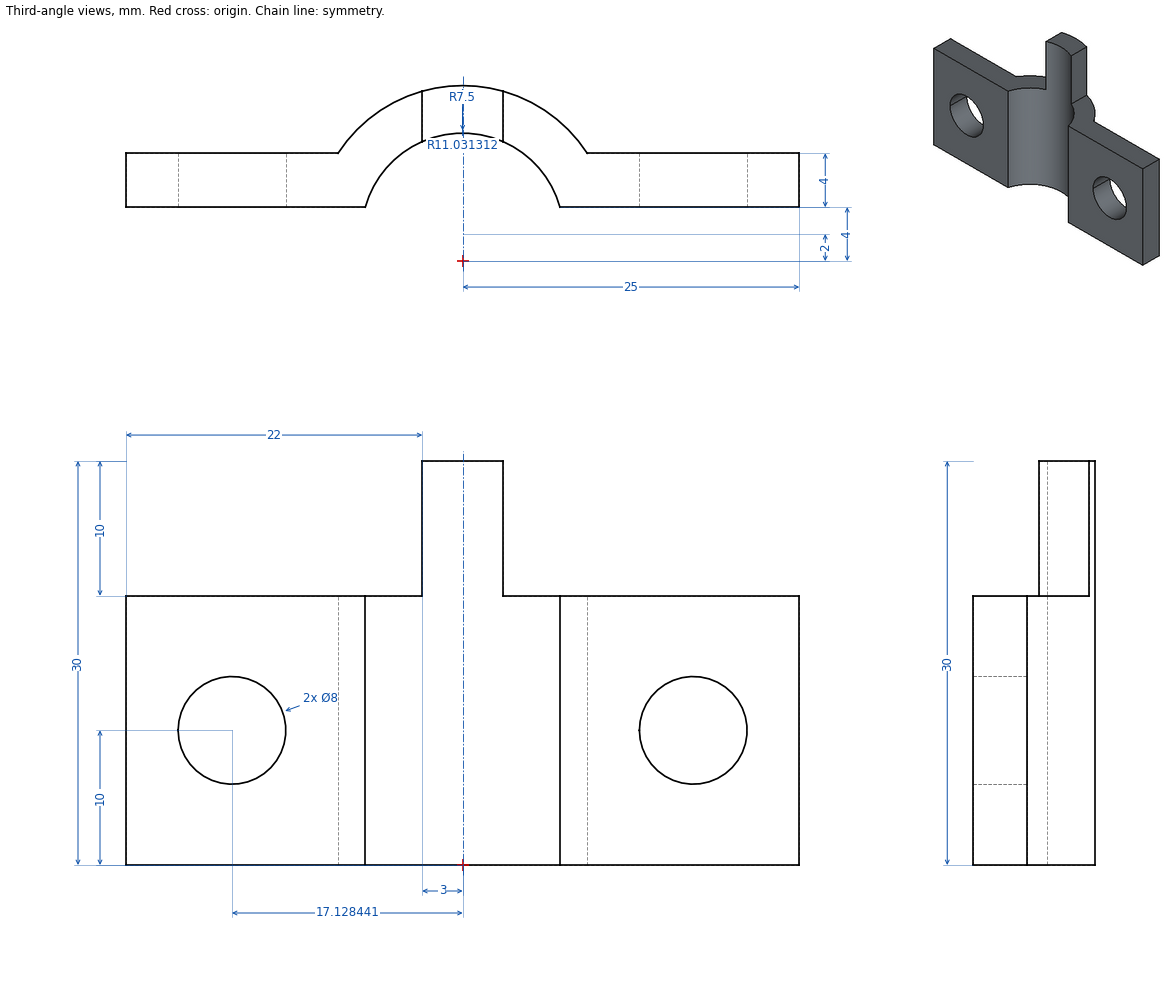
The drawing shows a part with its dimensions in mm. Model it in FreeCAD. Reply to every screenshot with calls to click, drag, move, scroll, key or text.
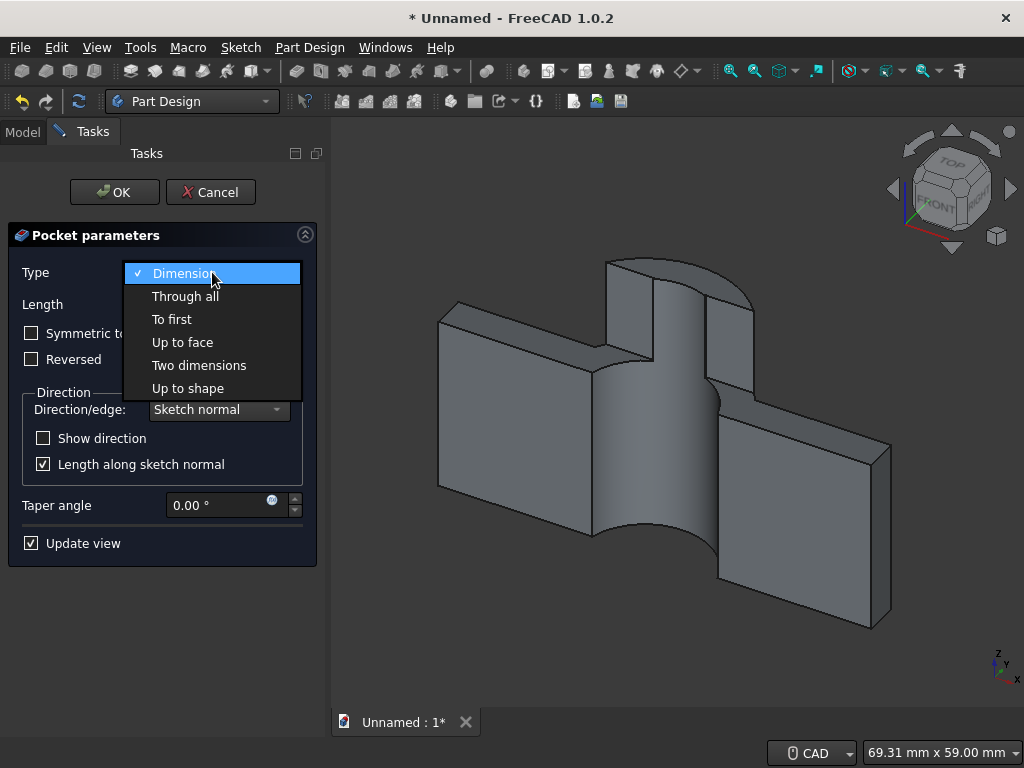
click(212, 296)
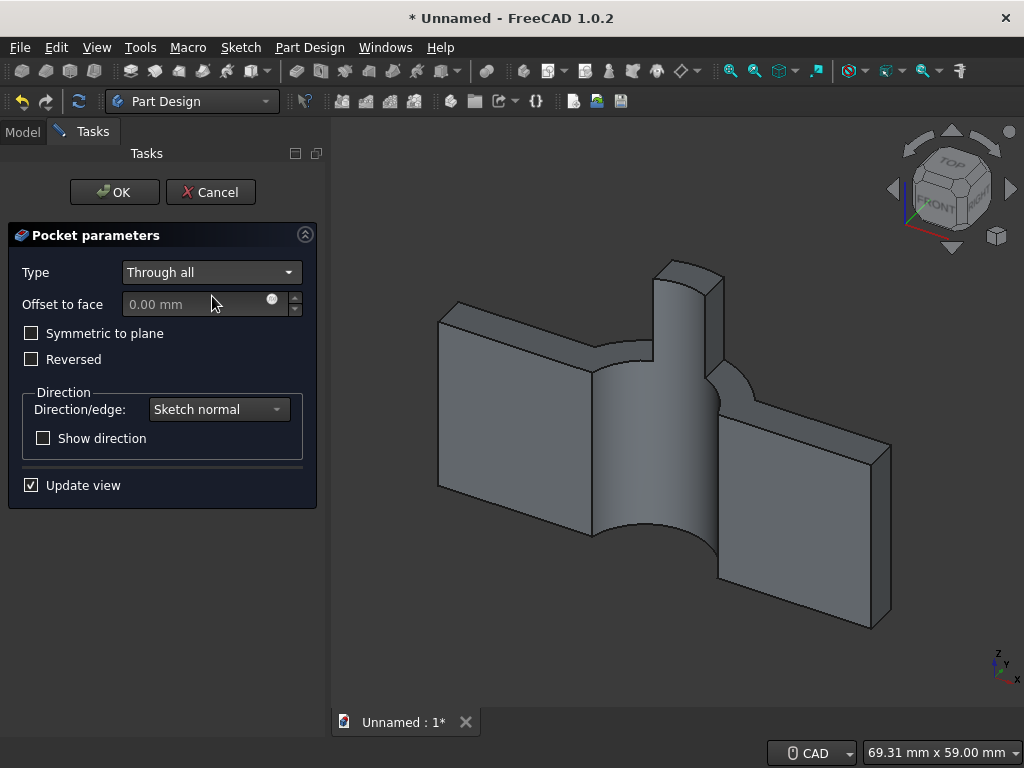
click(115, 192)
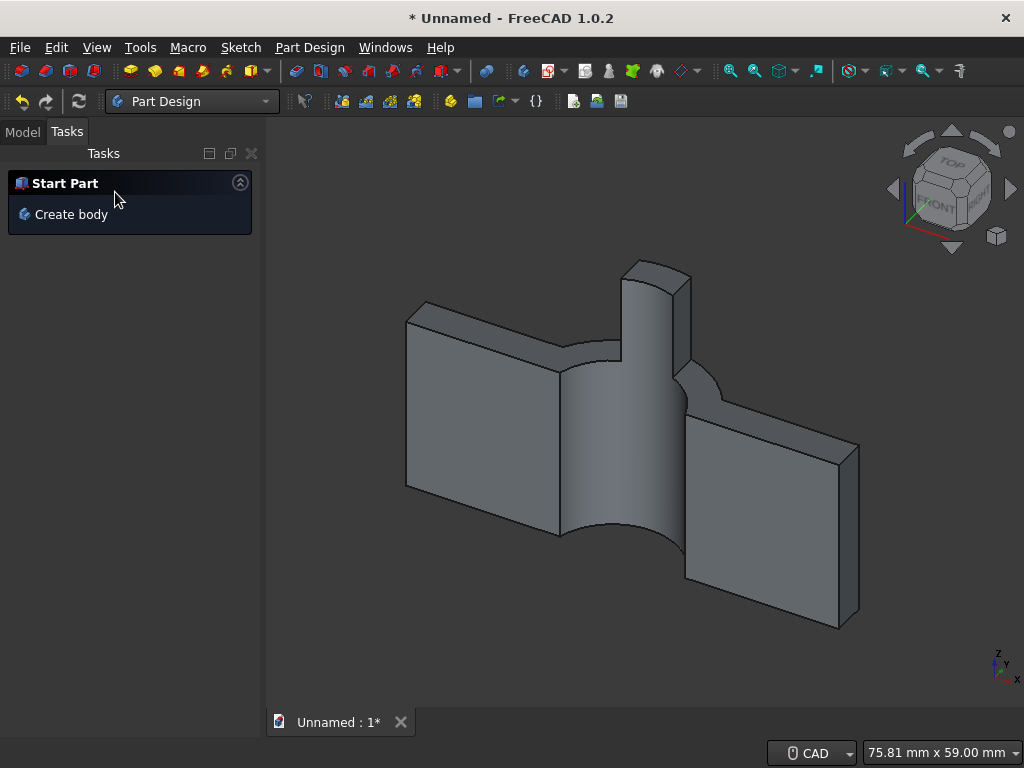
key(4)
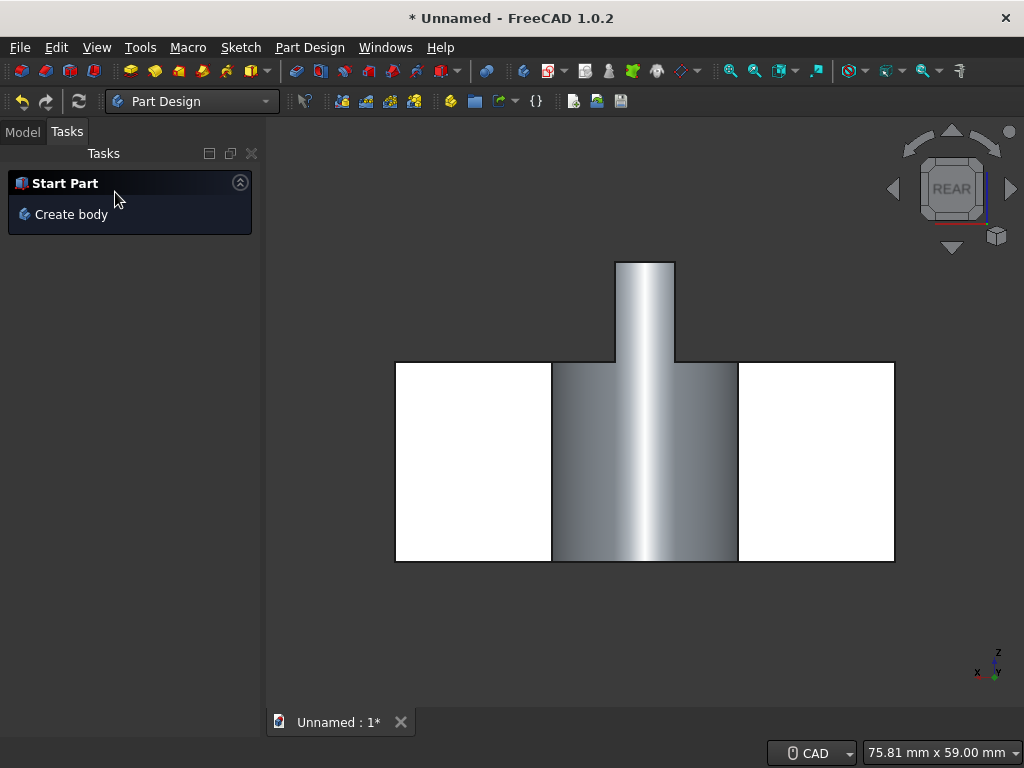
click(816, 461)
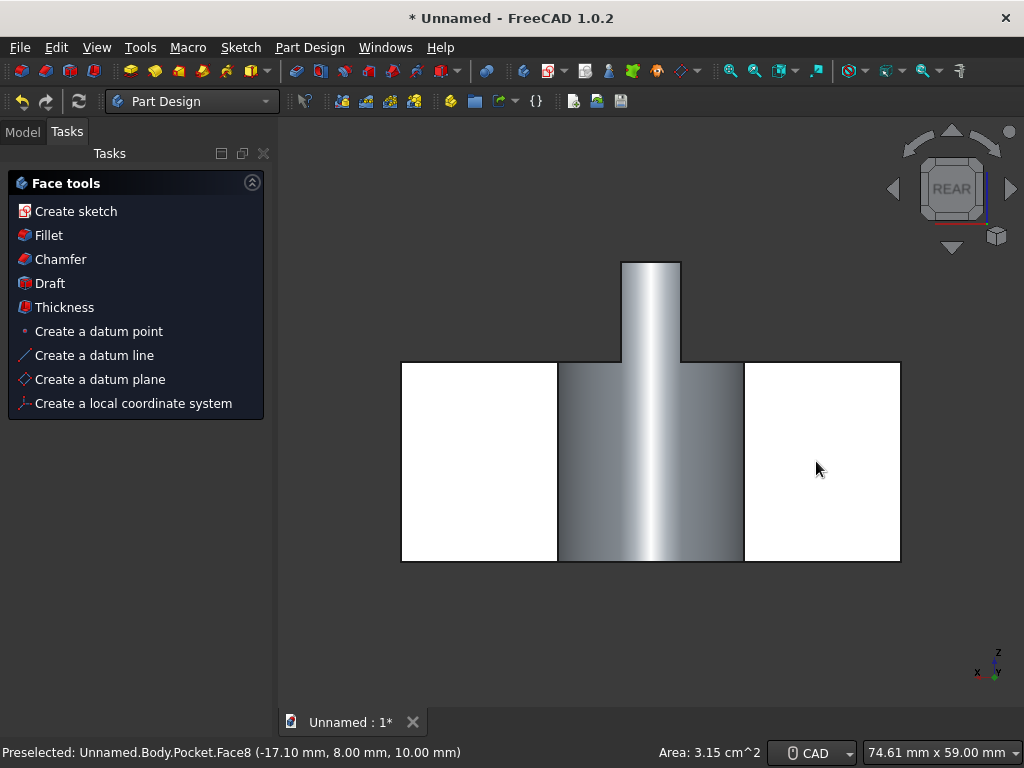
click(548, 72)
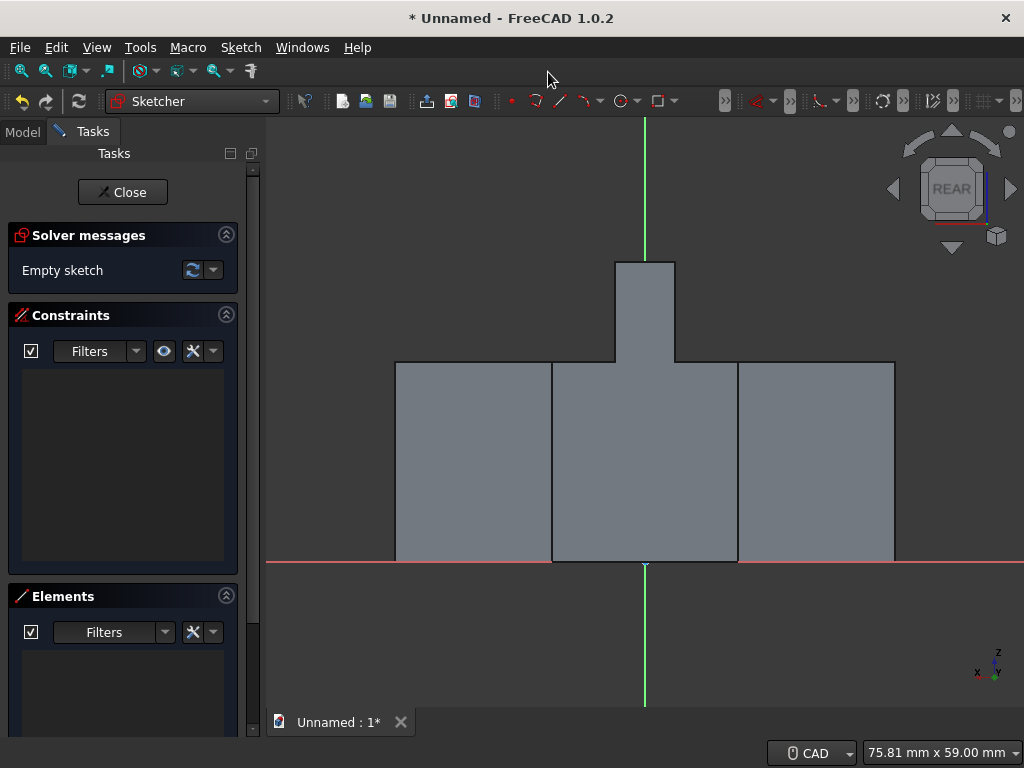
scroll(294, 145, down, 1)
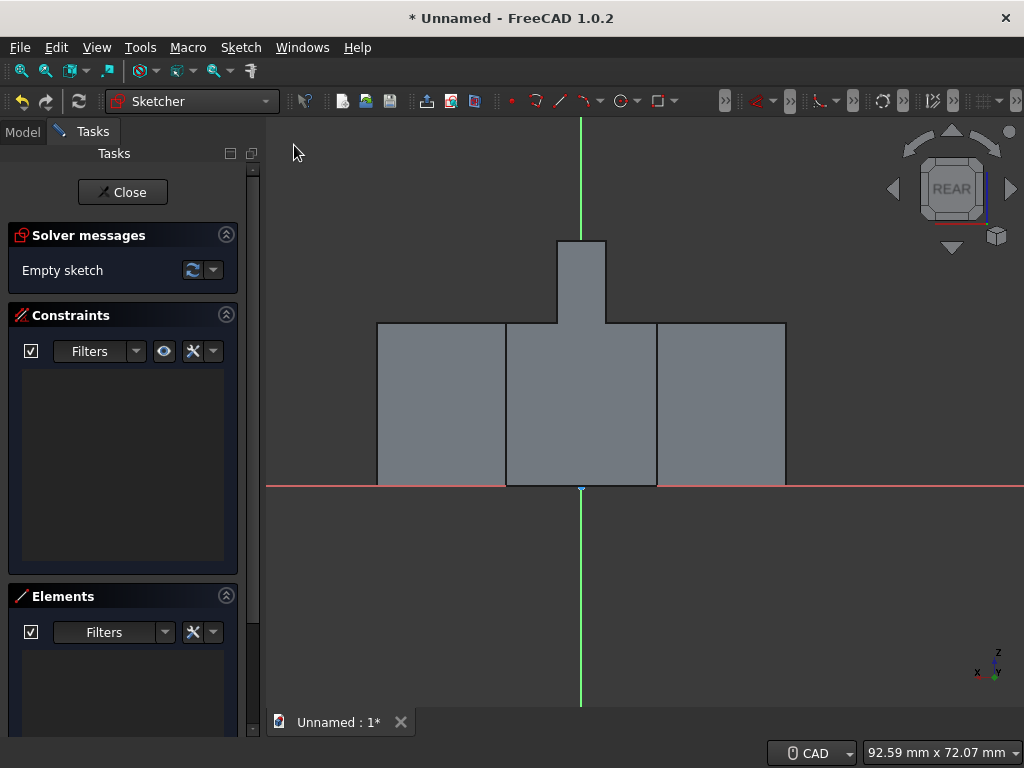
click(622, 102)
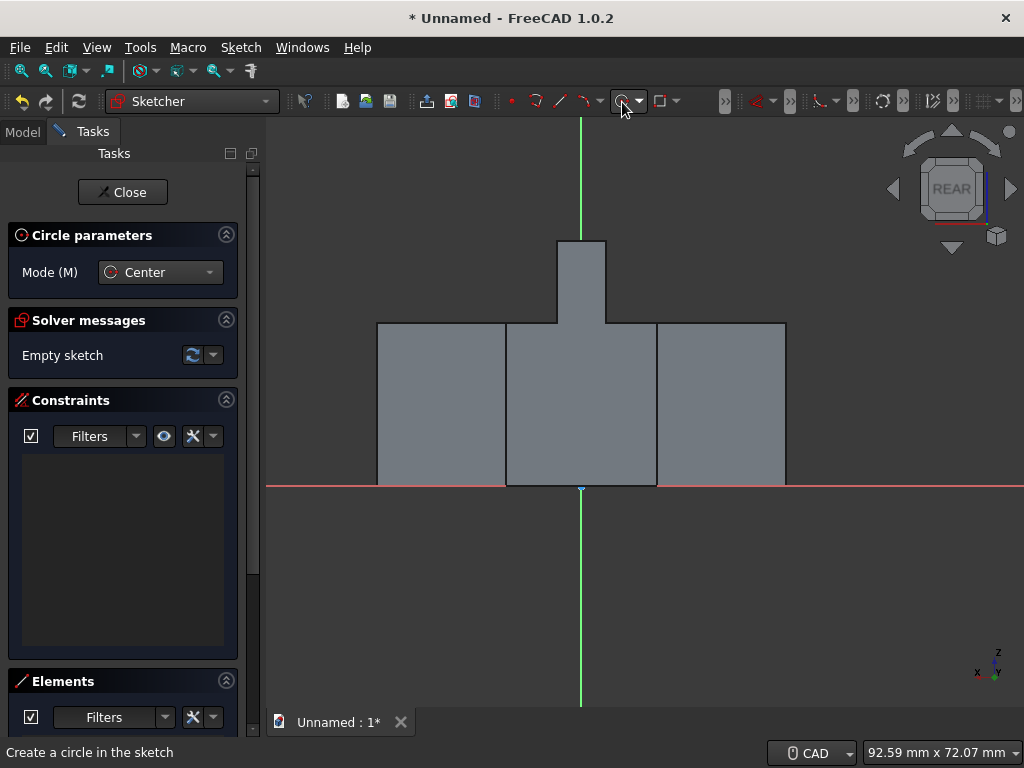
click(722, 405)
click(745, 381)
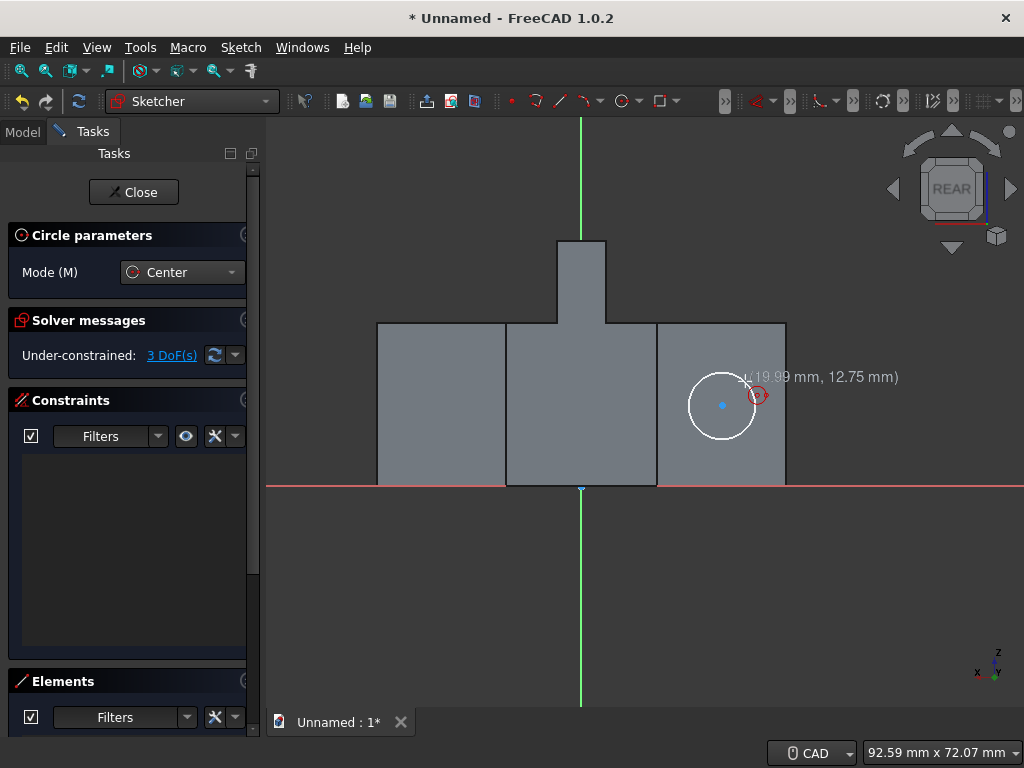
click(441, 405)
click(464, 381)
key(Escape)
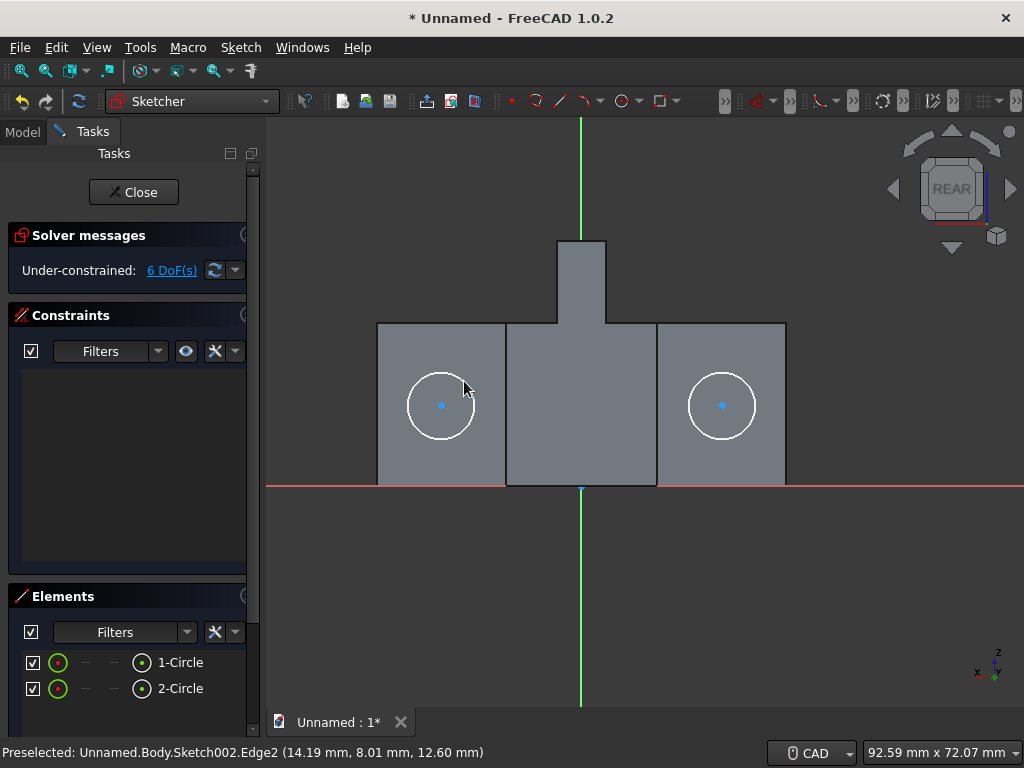
click(745, 382)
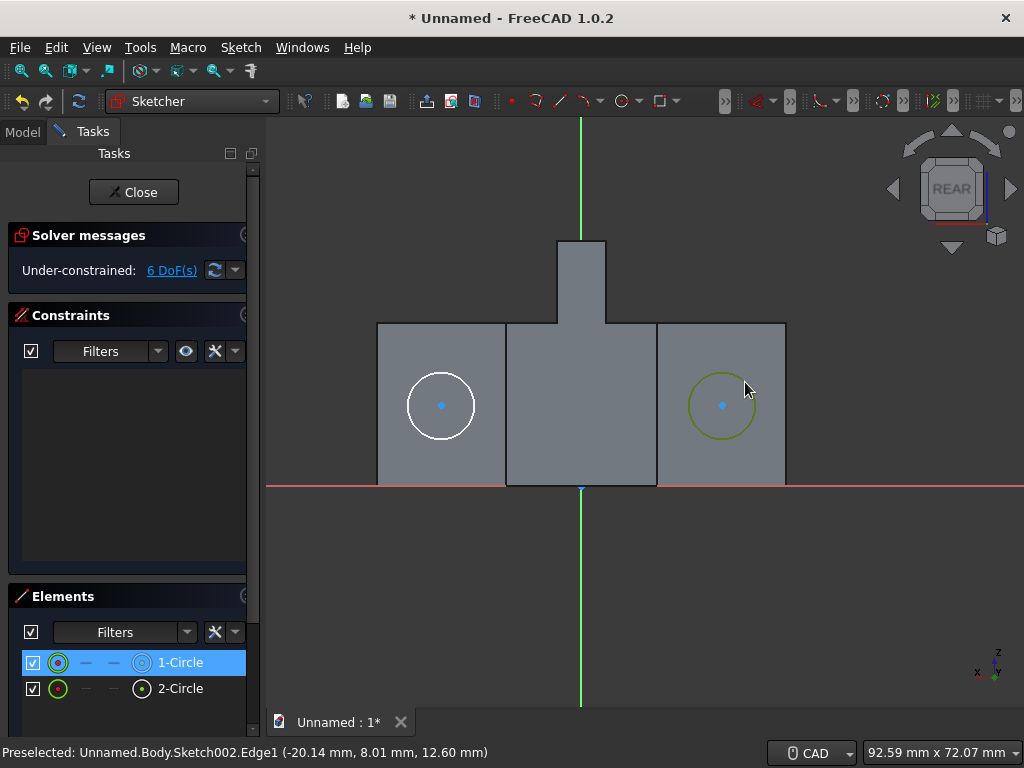
click(464, 382)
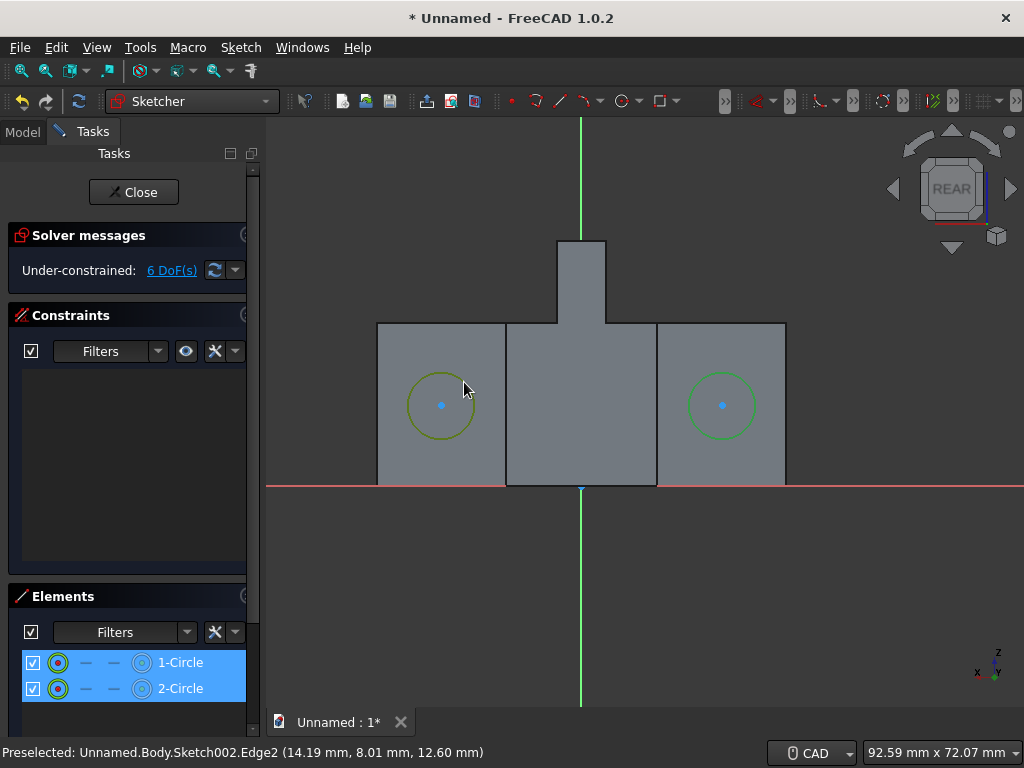
key(e)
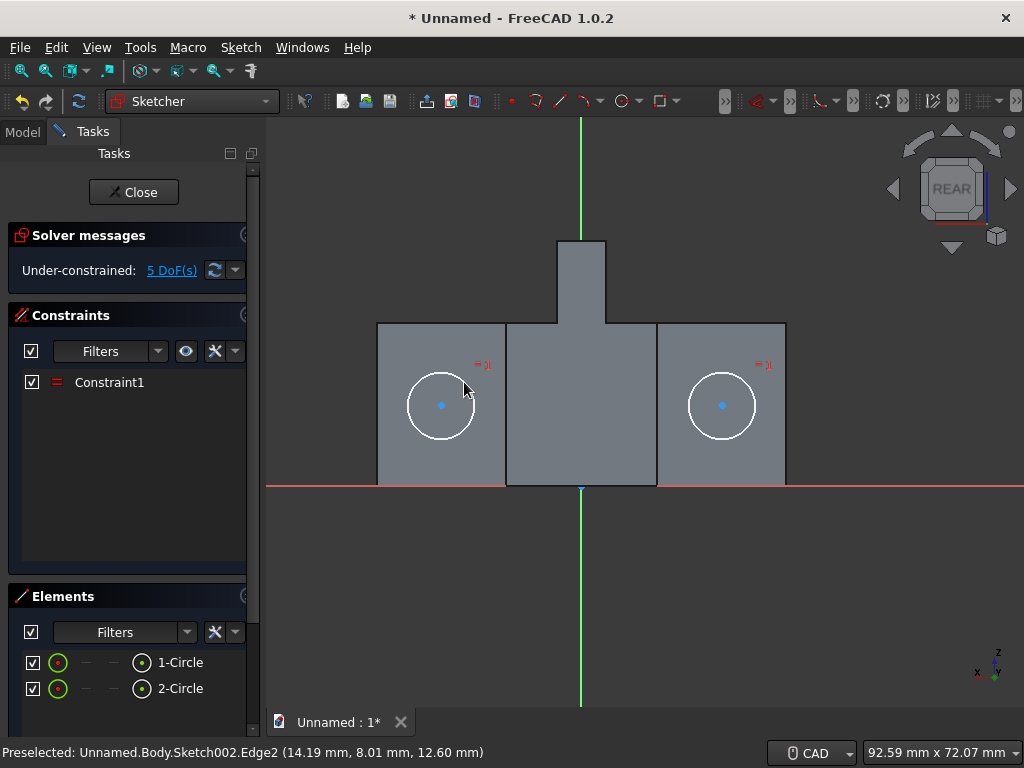
click(722, 406)